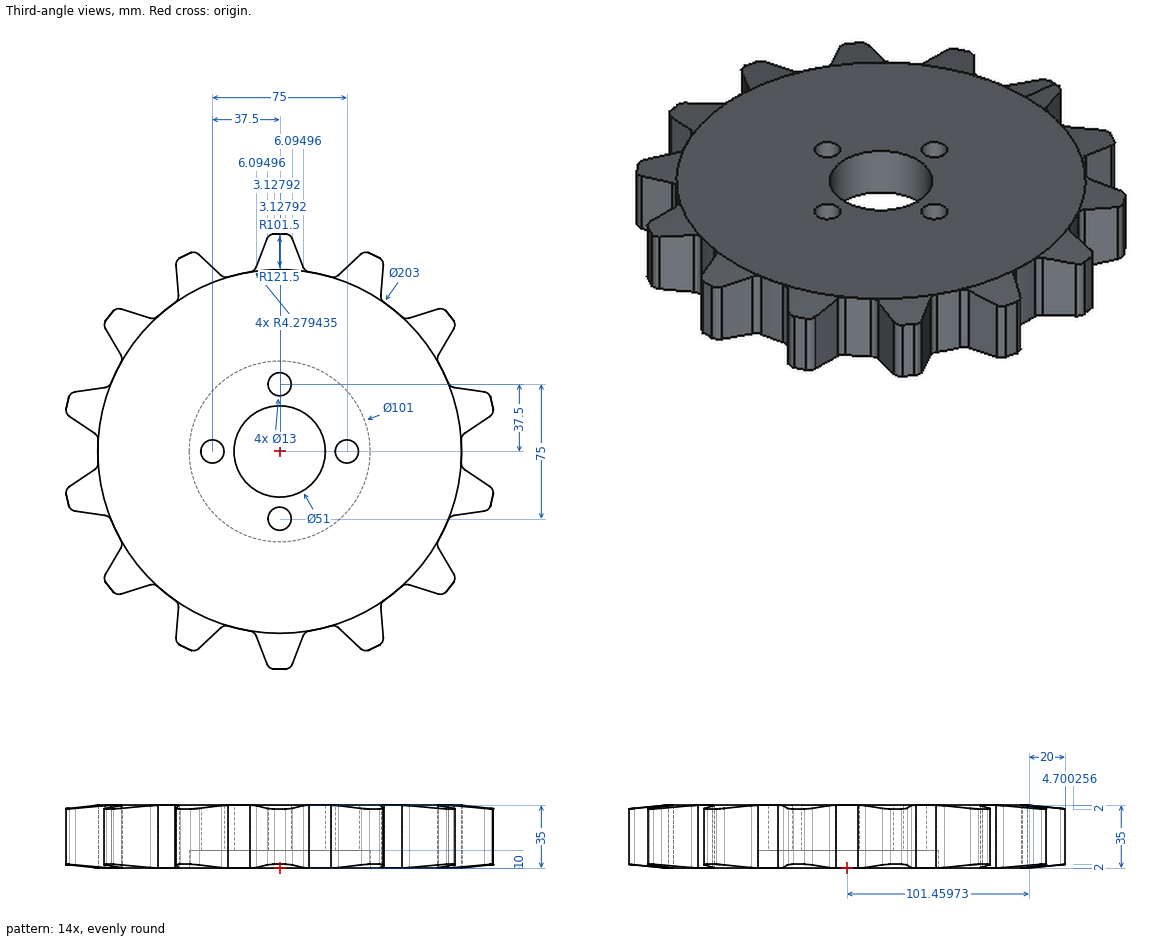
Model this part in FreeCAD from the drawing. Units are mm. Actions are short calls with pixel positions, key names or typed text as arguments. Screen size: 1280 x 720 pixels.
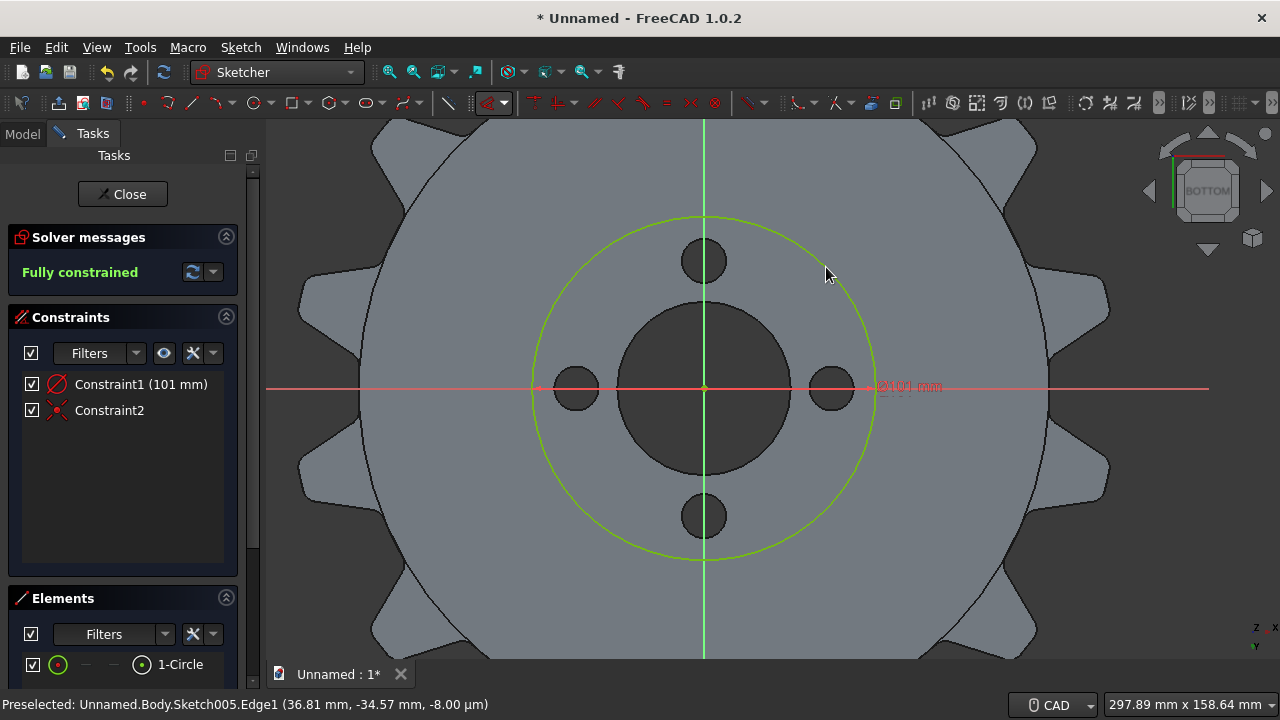
click(123, 194)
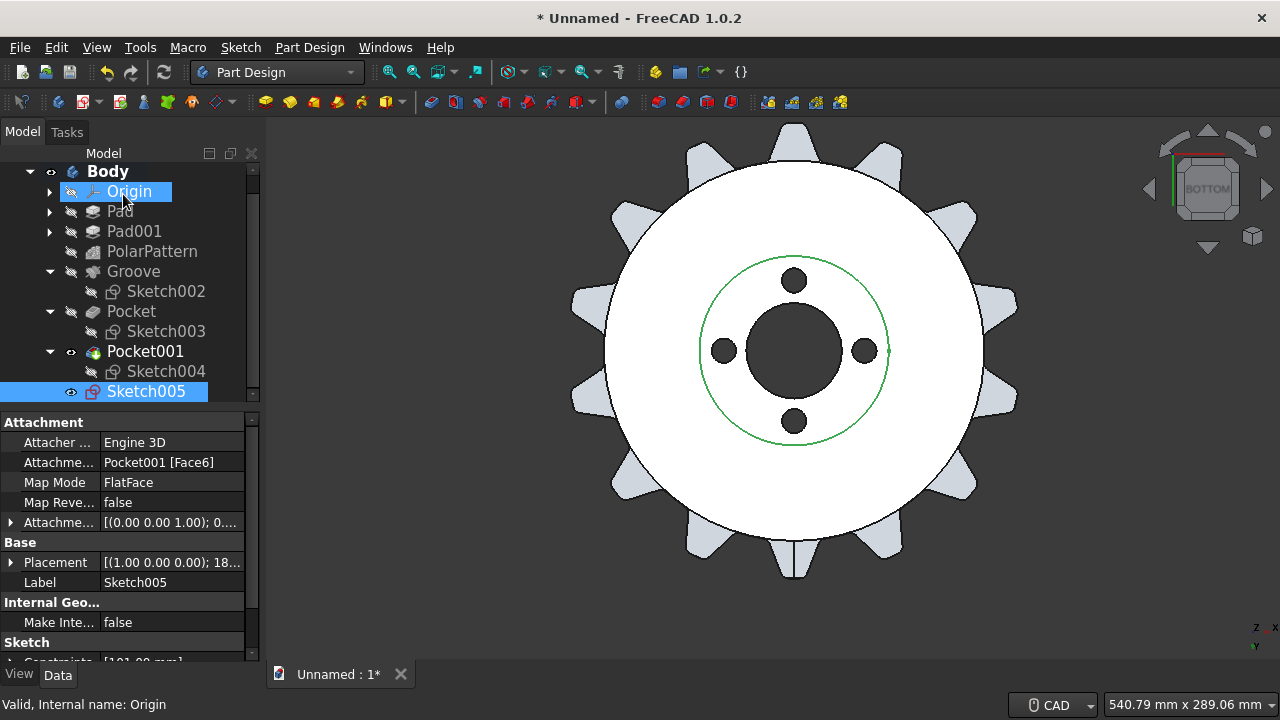
click(432, 102)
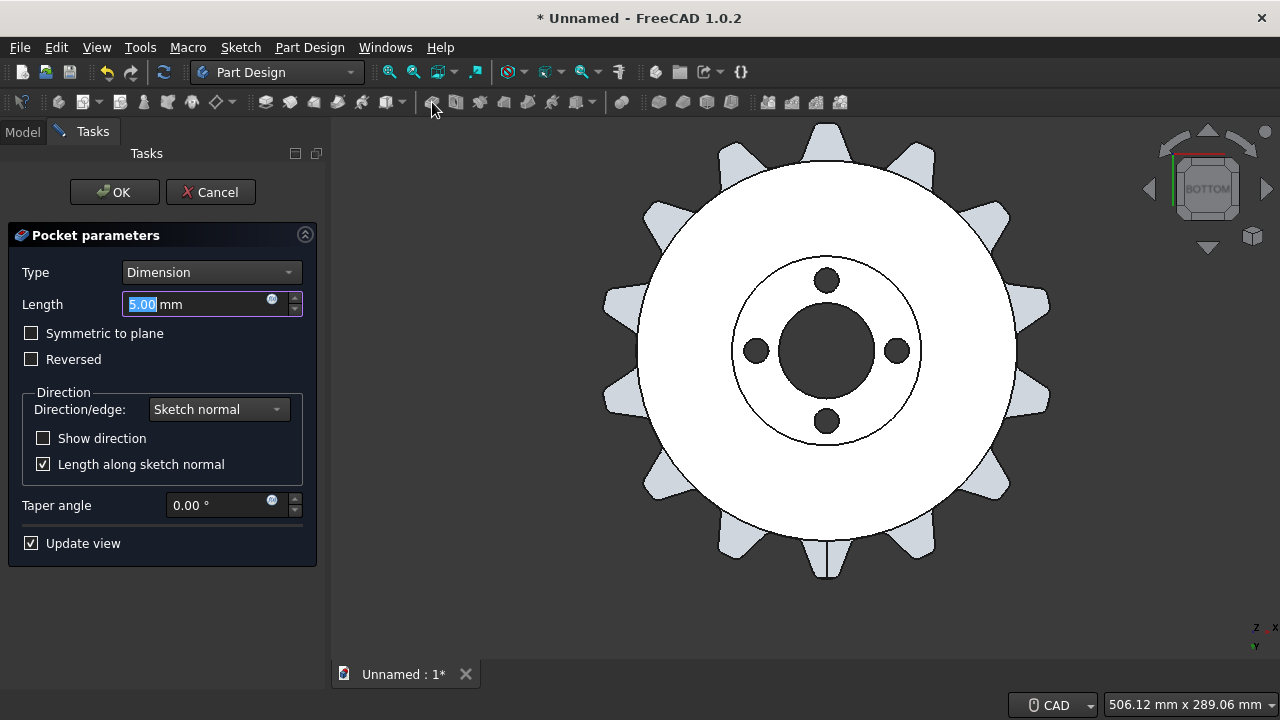
text(10)
key(Tab)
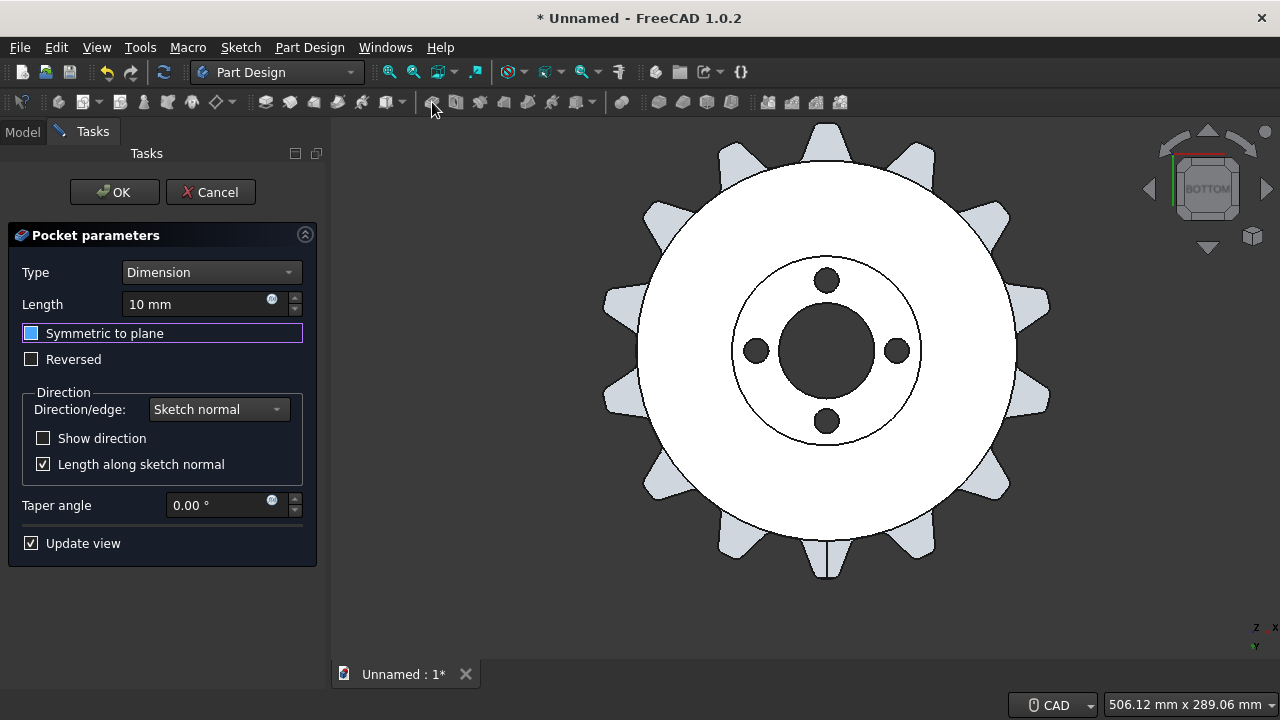
click(115, 192)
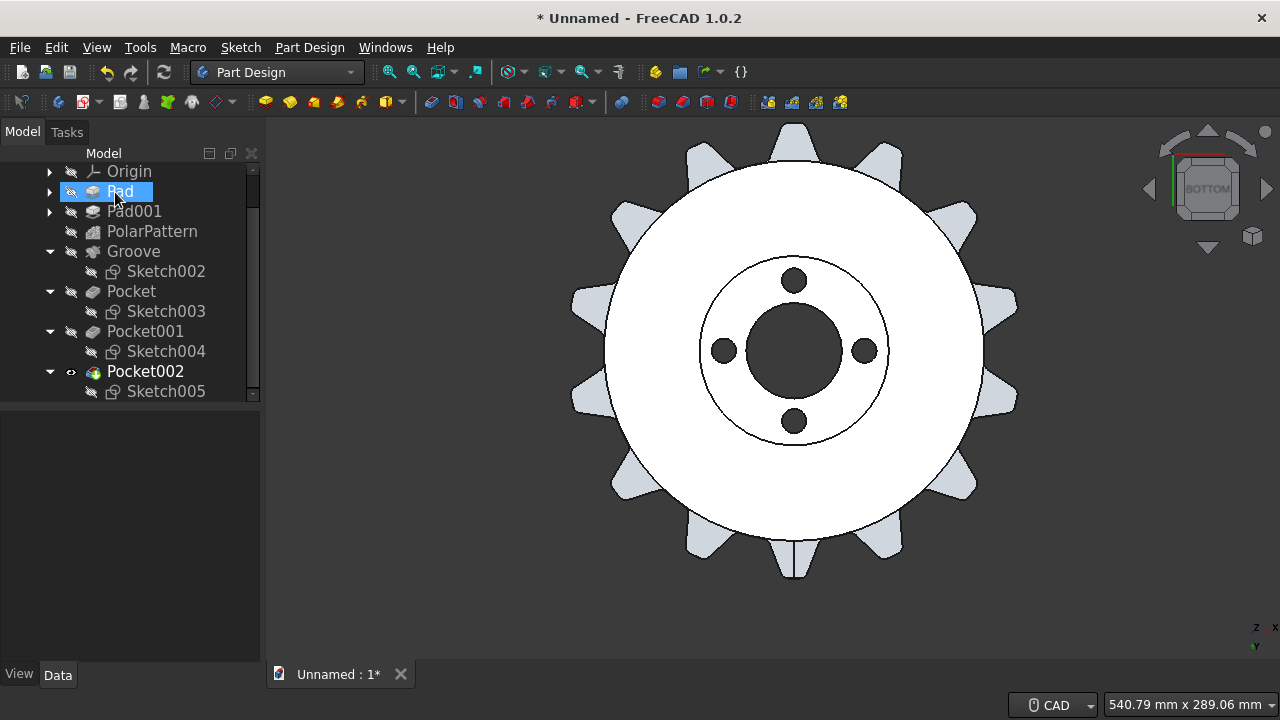
key(0)